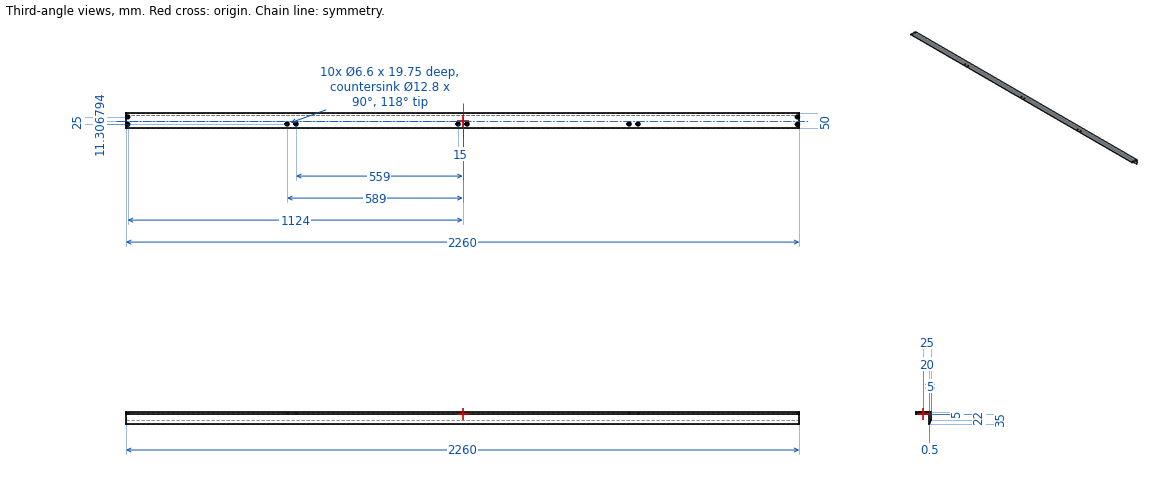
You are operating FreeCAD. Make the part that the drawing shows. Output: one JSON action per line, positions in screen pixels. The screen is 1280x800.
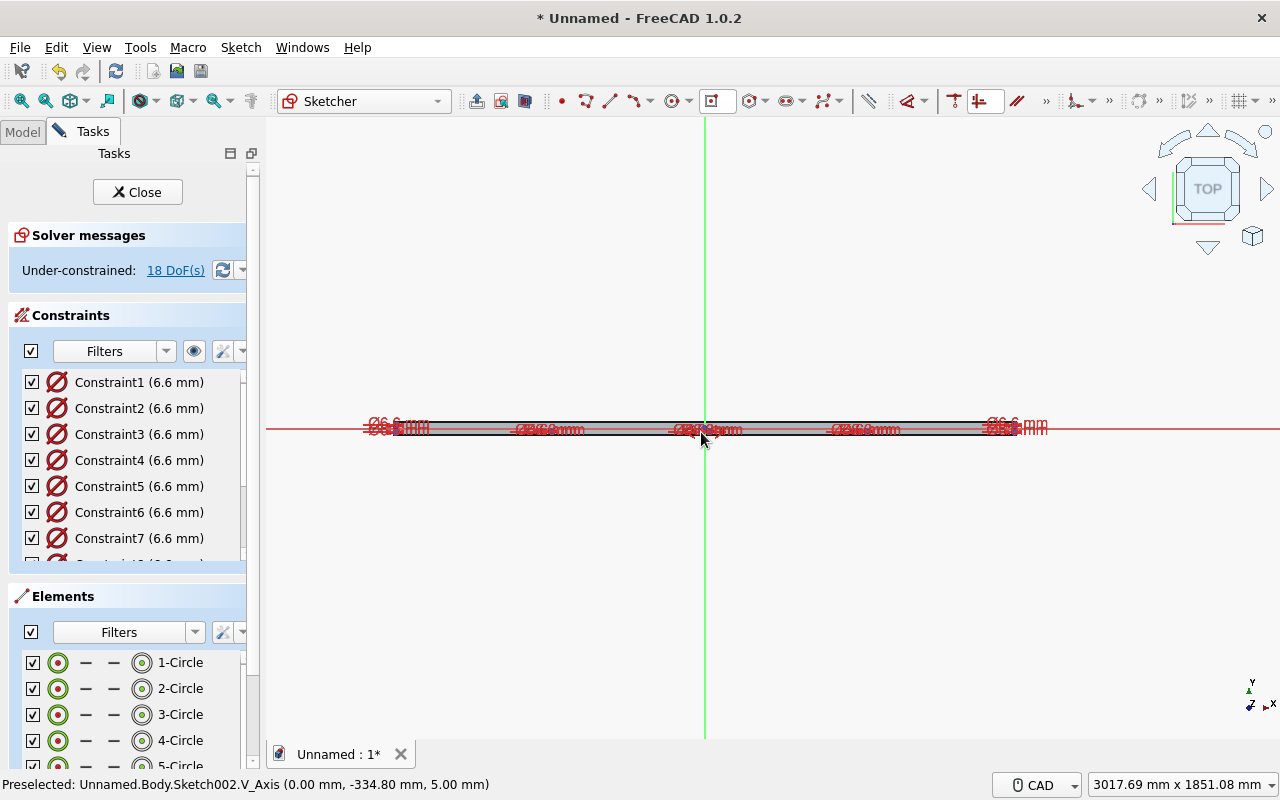
{"action": "scroll", "coordinate": [551, 432], "scroll_direction": "up", "scroll_amount": 2}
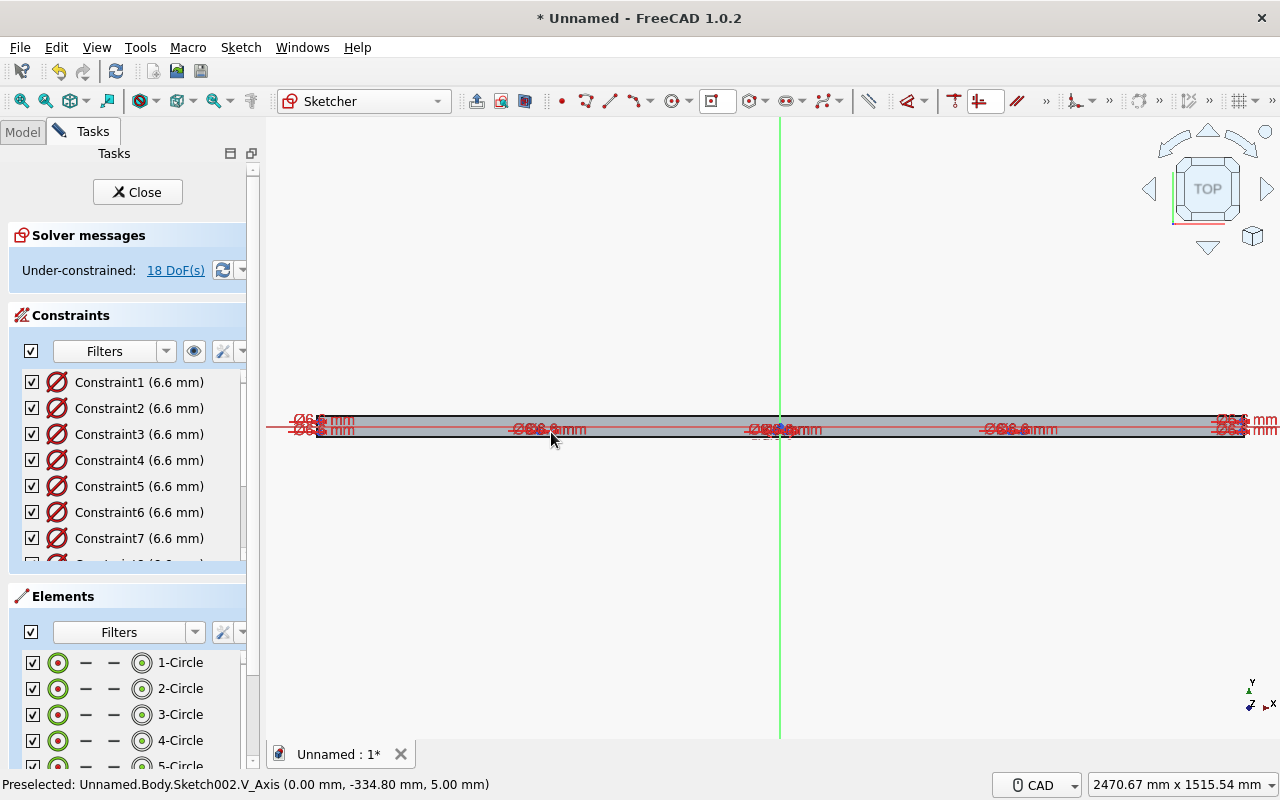
{"action": "left_click", "coordinate": [551, 431]}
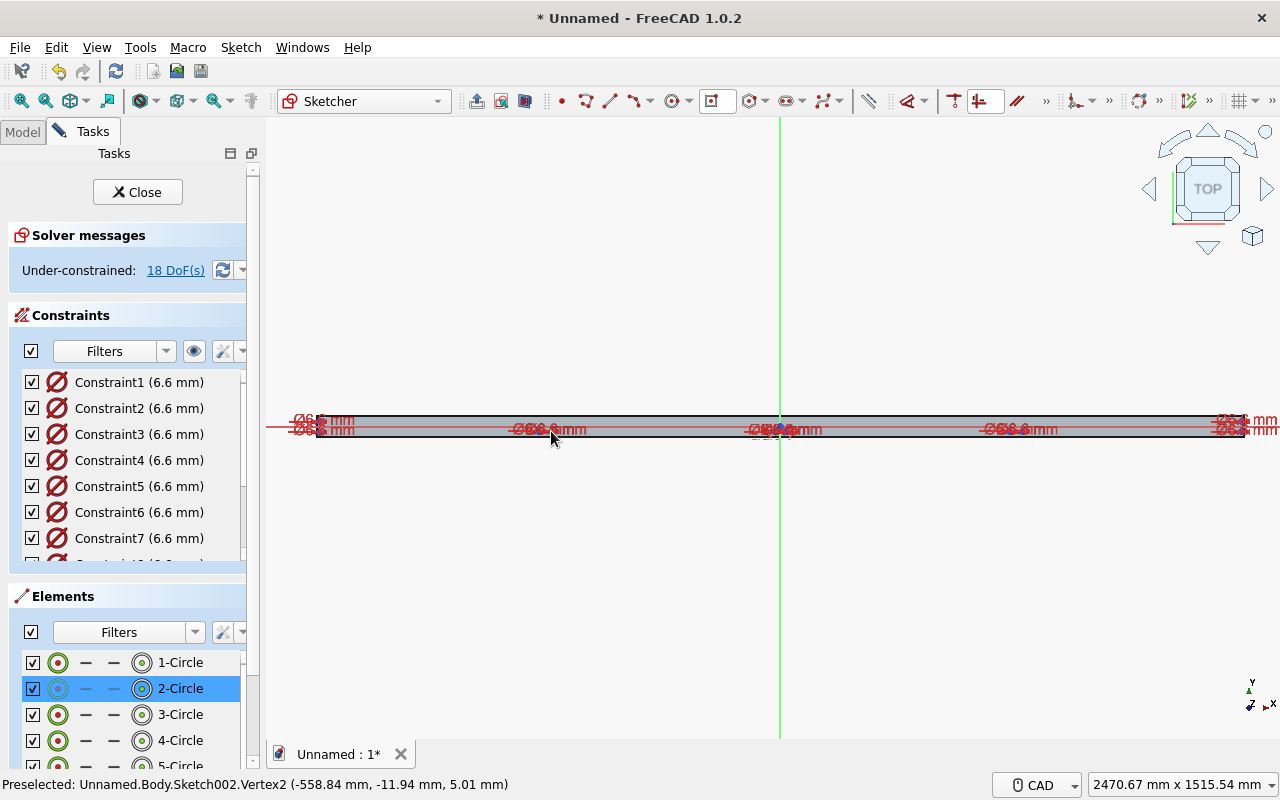
{"action": "left_click", "coordinate": [1010, 431]}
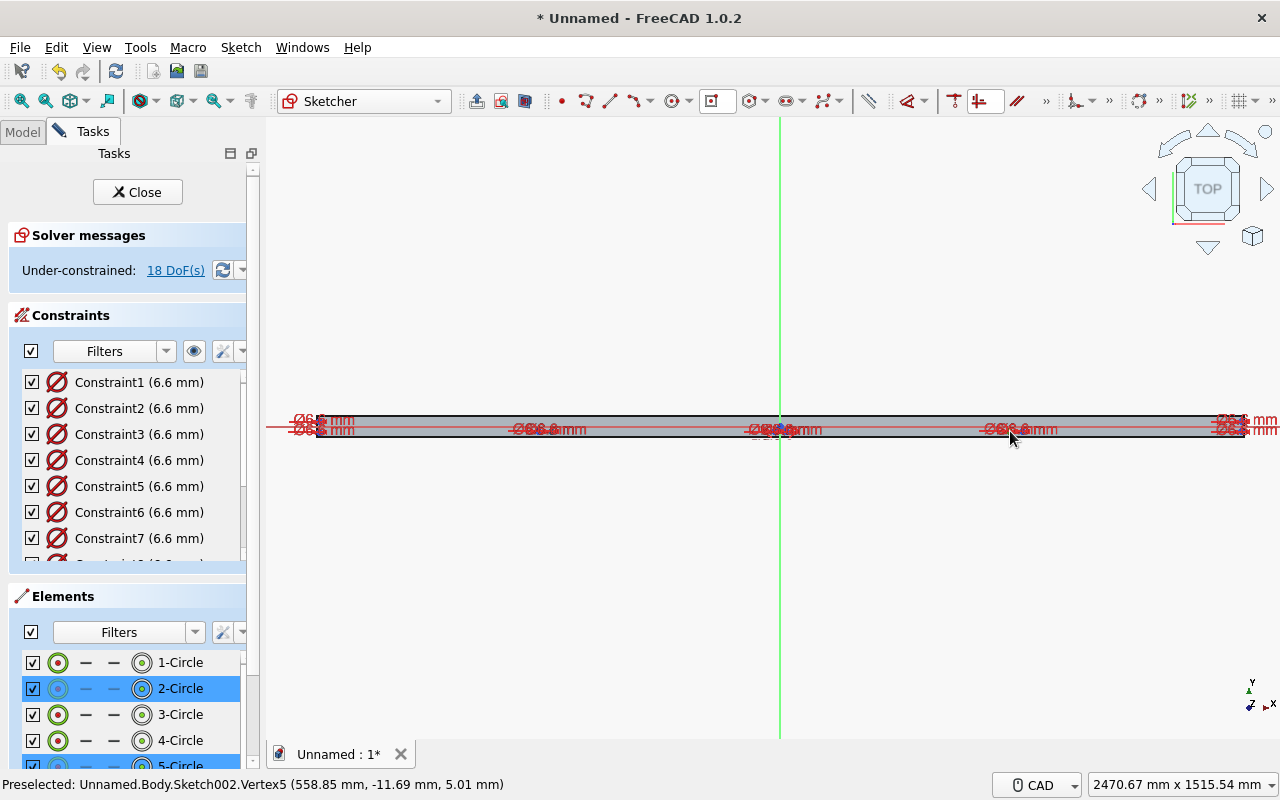
{"action": "left_click", "coordinate": [780, 671]}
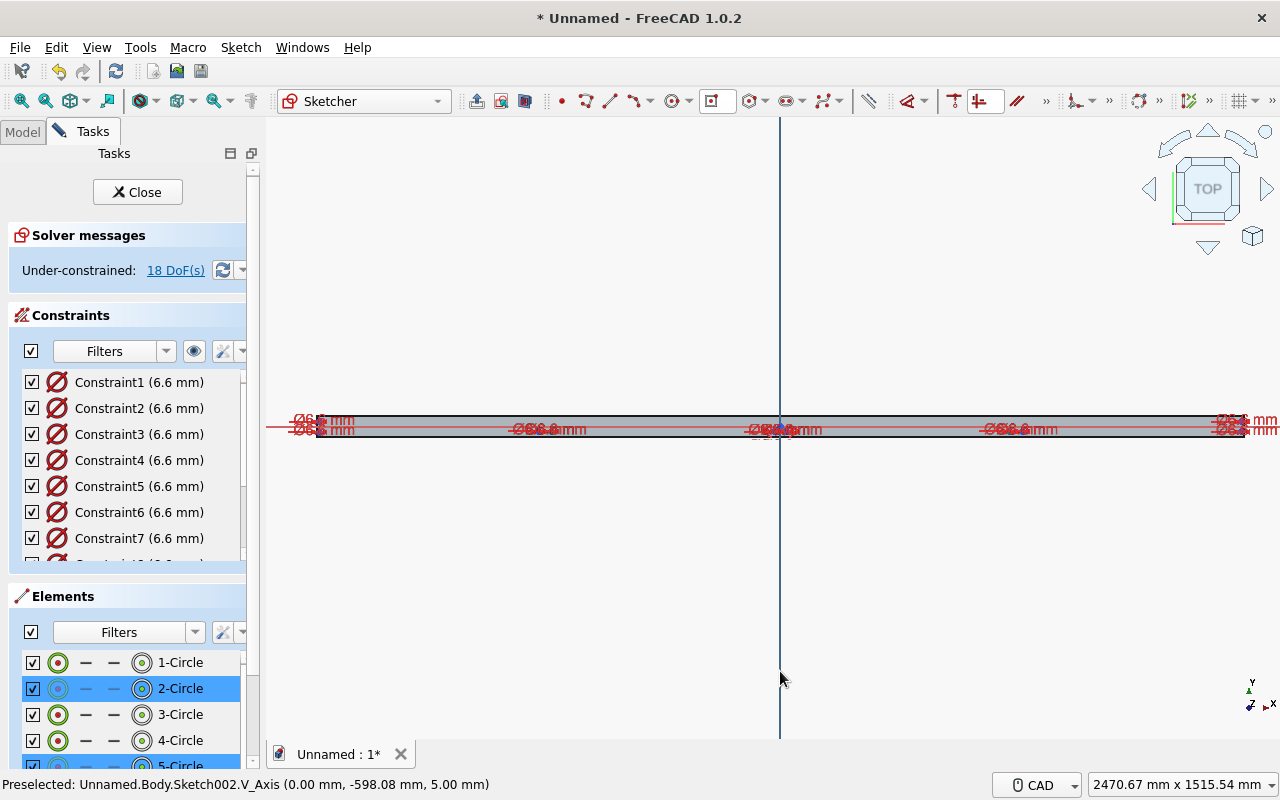
{"action": "key", "text": "s"}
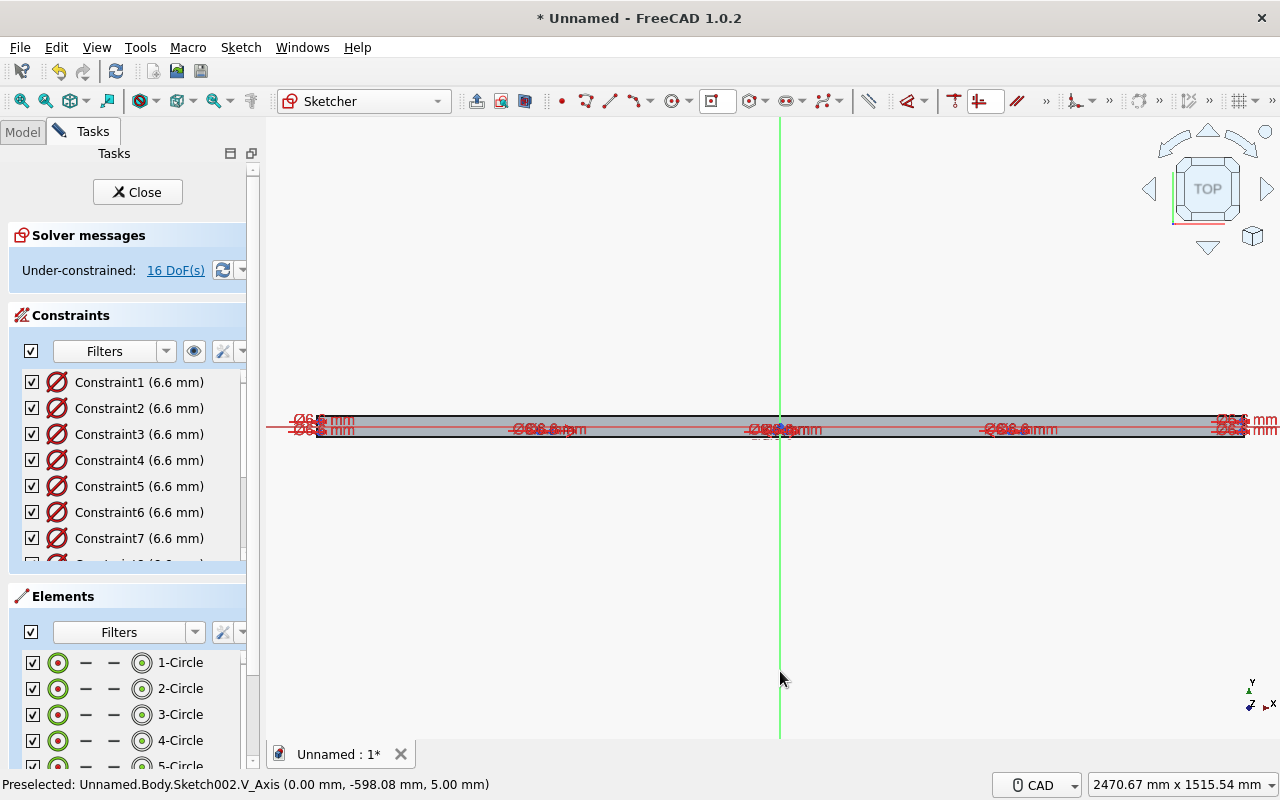
{"action": "left_click", "coordinate": [539, 431]}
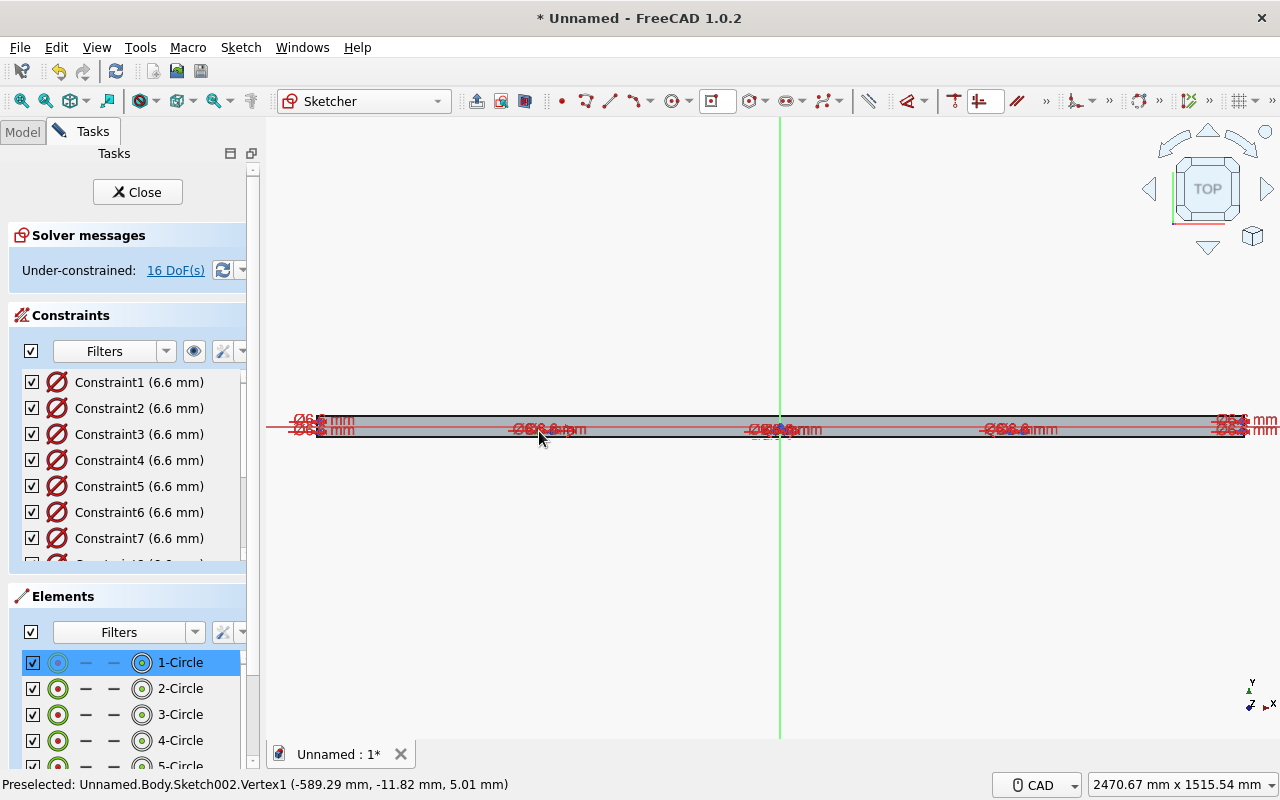
{"action": "left_click", "coordinate": [1022, 431]}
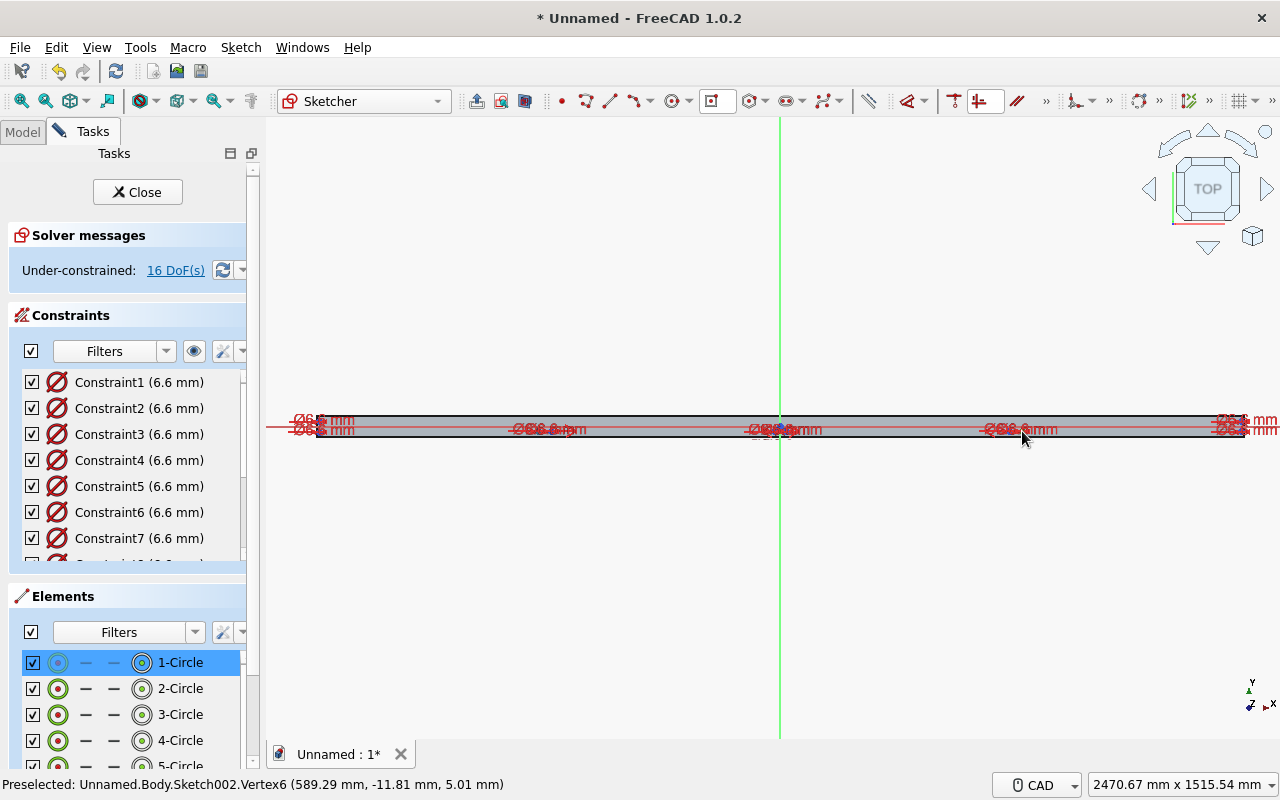
{"action": "left_click", "coordinate": [780, 671]}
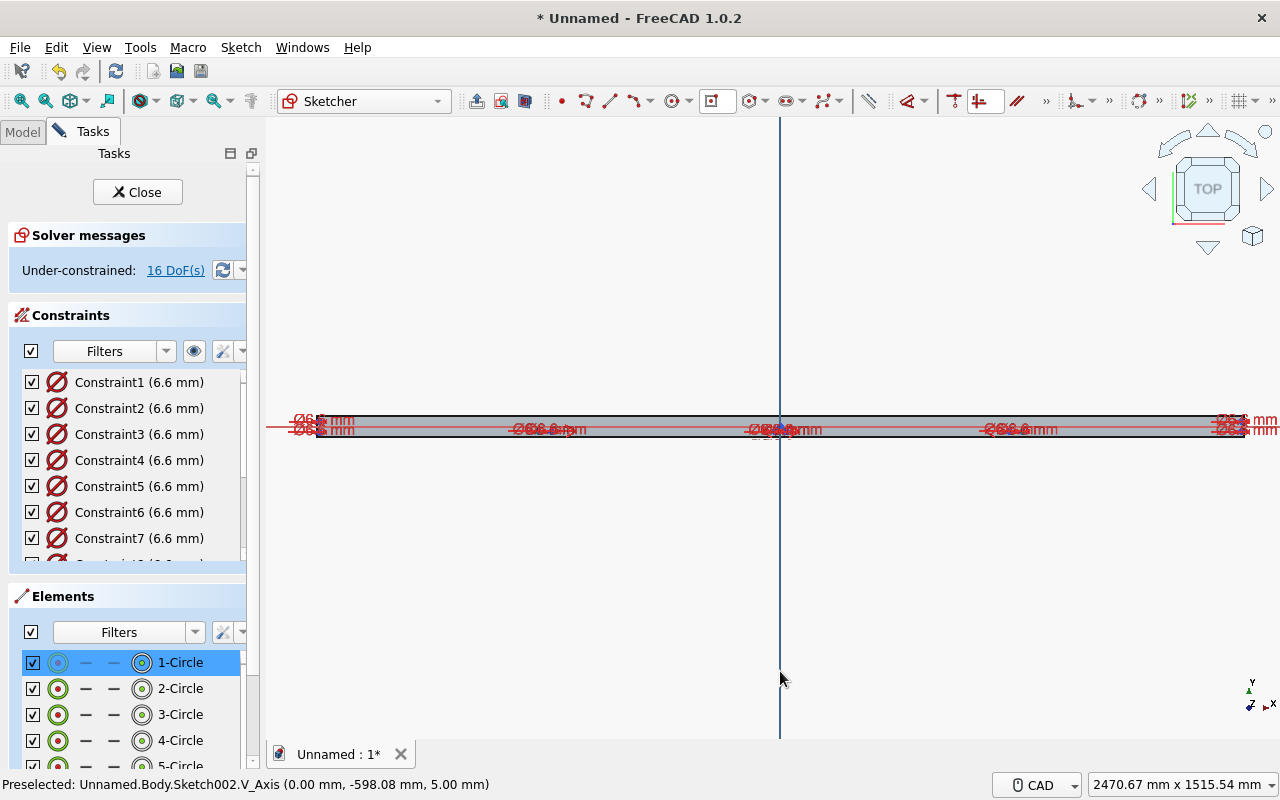
{"action": "key", "text": "s"}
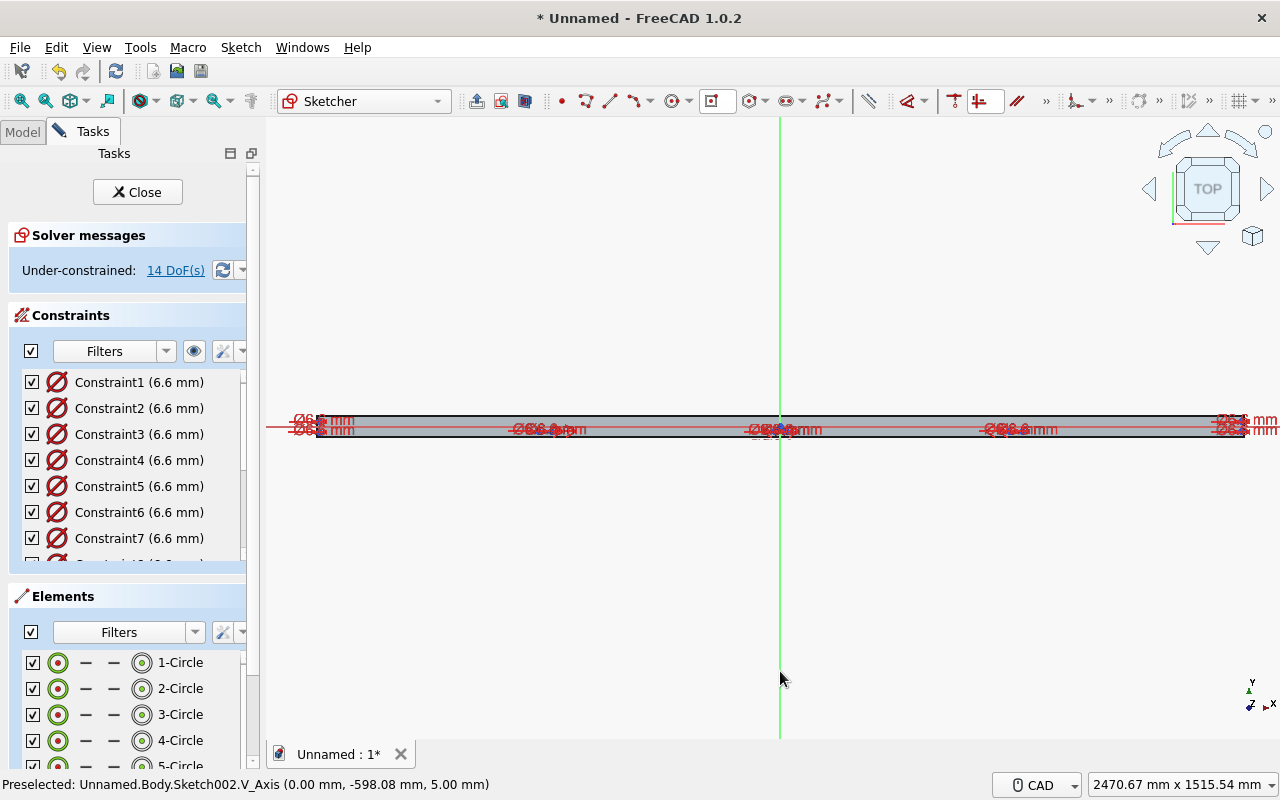
{"action": "left_click", "coordinate": [319, 432]}